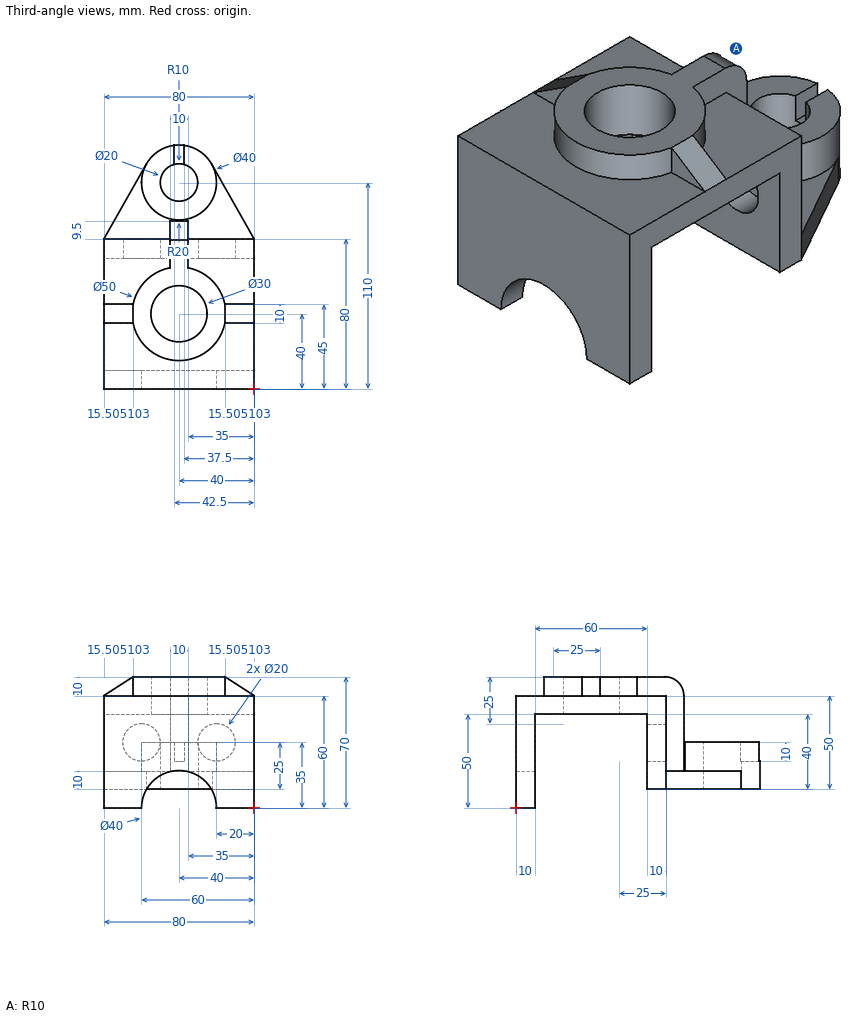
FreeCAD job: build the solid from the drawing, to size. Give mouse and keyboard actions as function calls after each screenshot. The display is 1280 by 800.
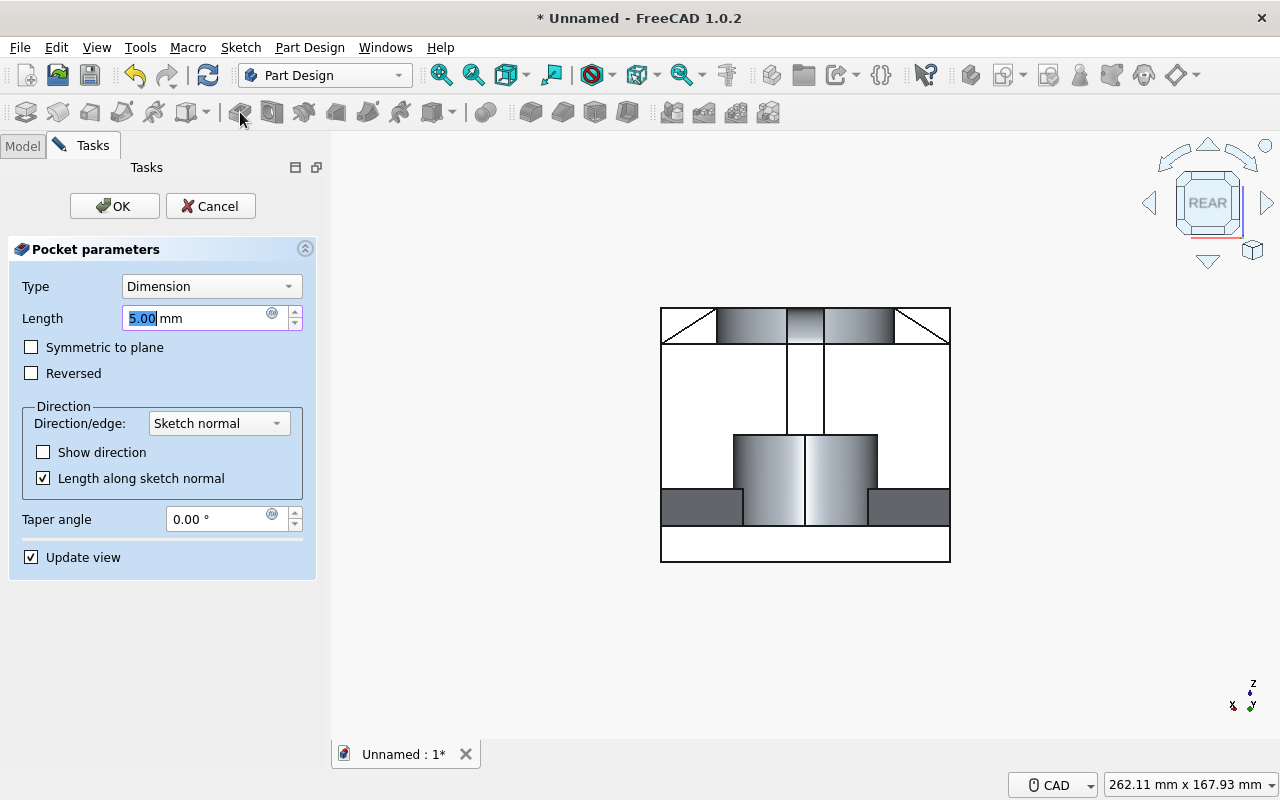
text(25)
key(Tab)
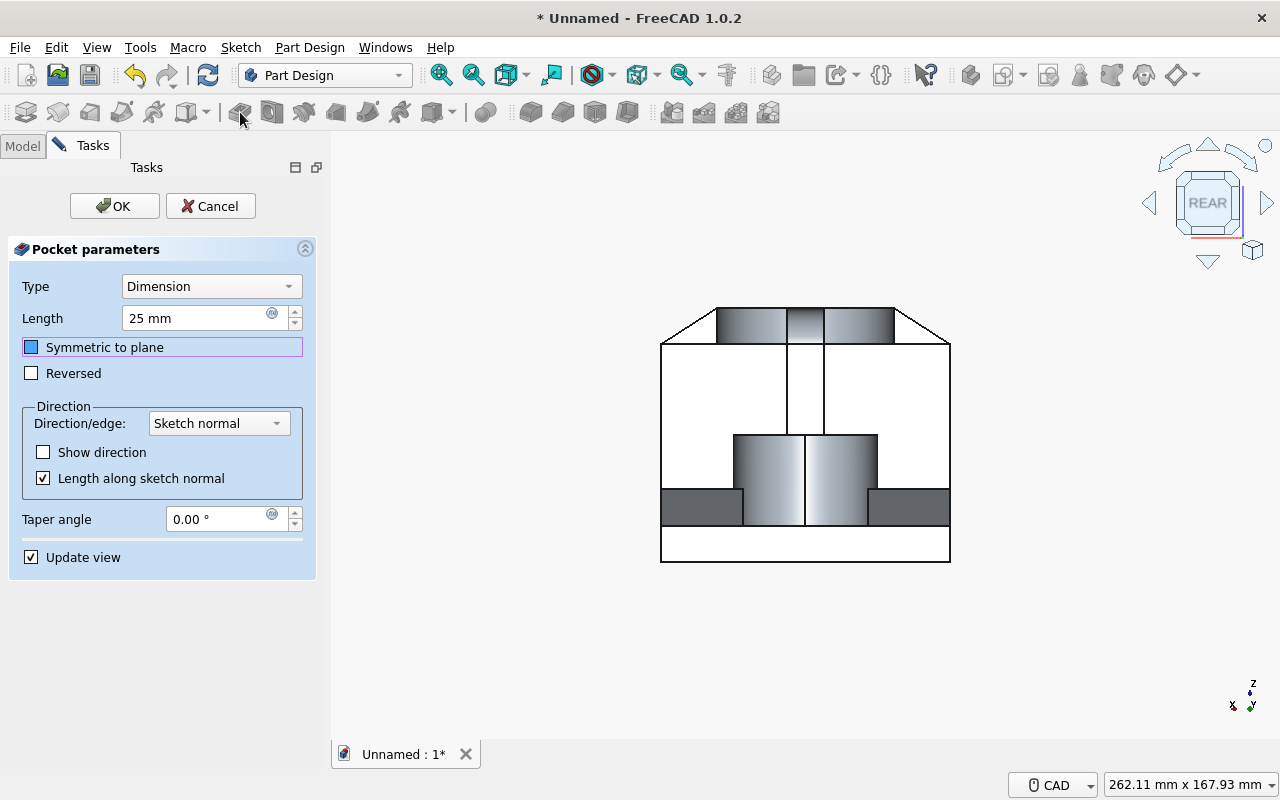
click(115, 206)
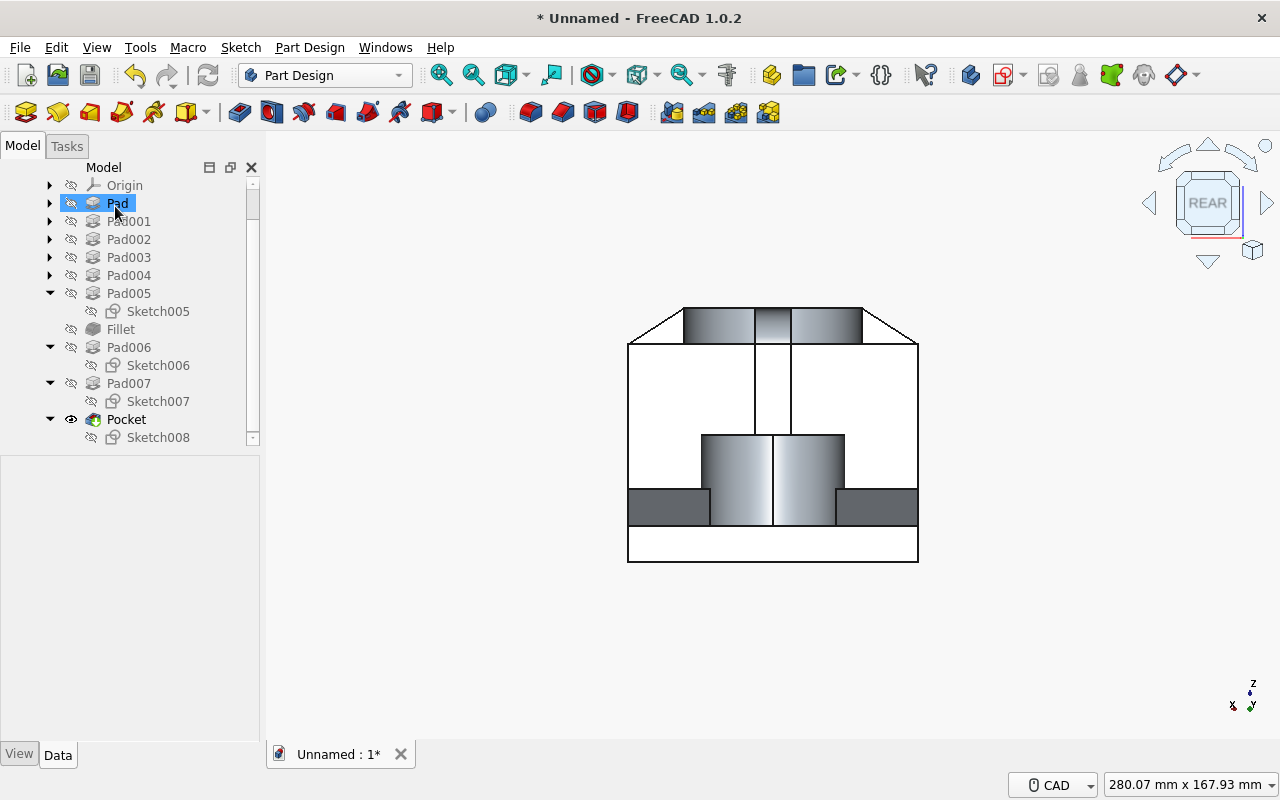
click(442, 76)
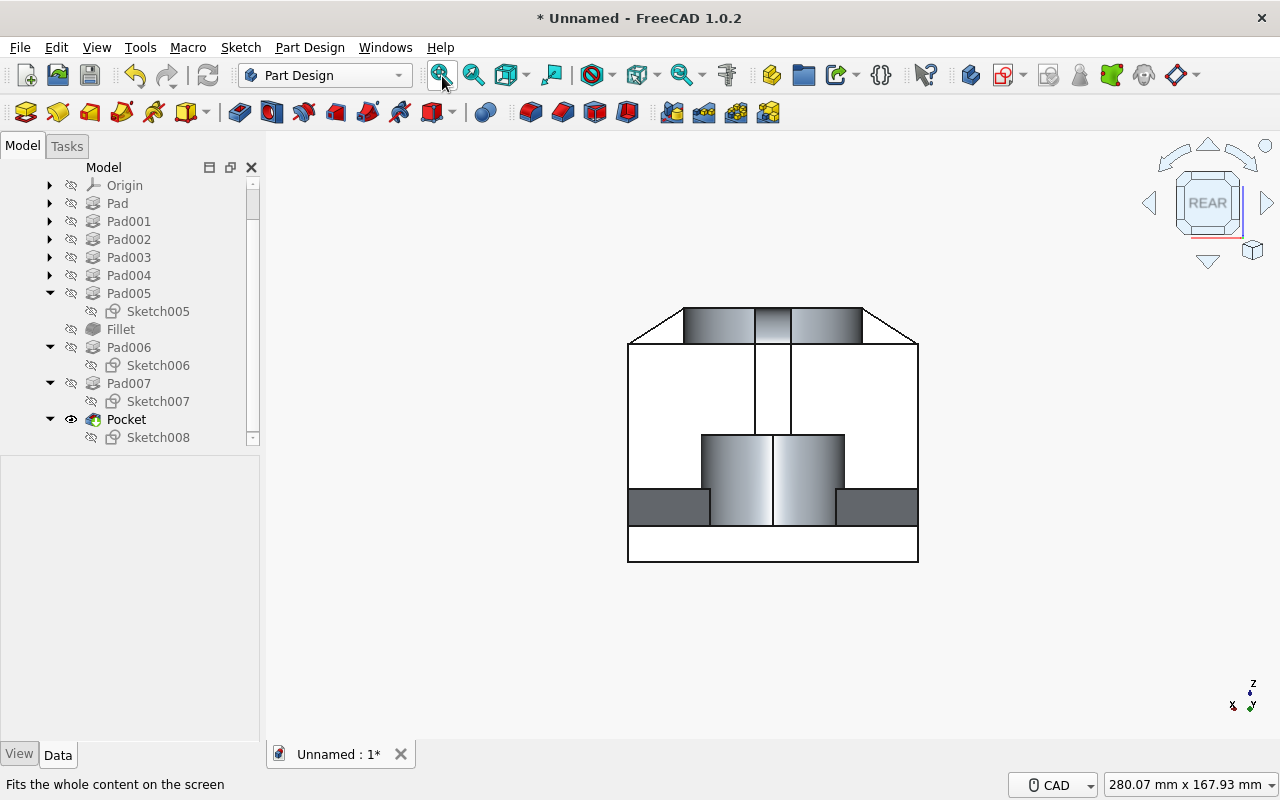
key(0)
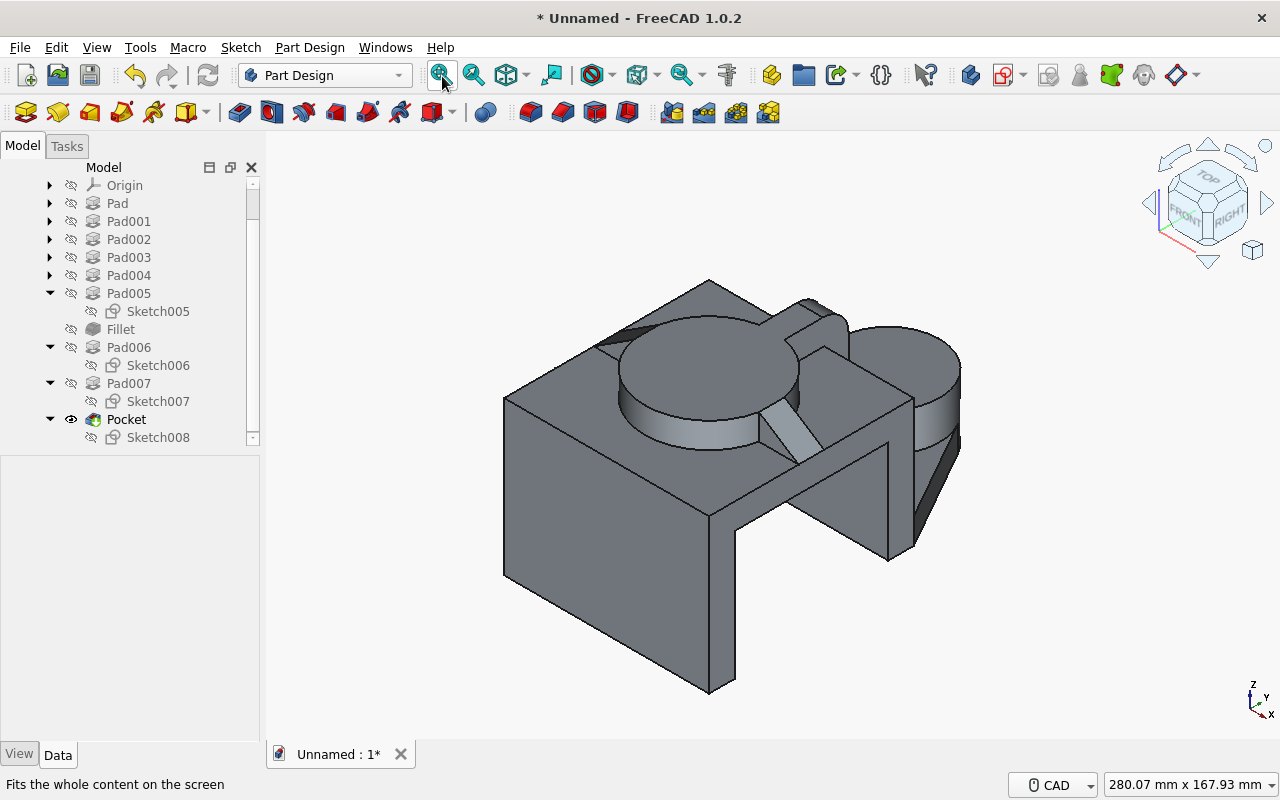
click(704, 370)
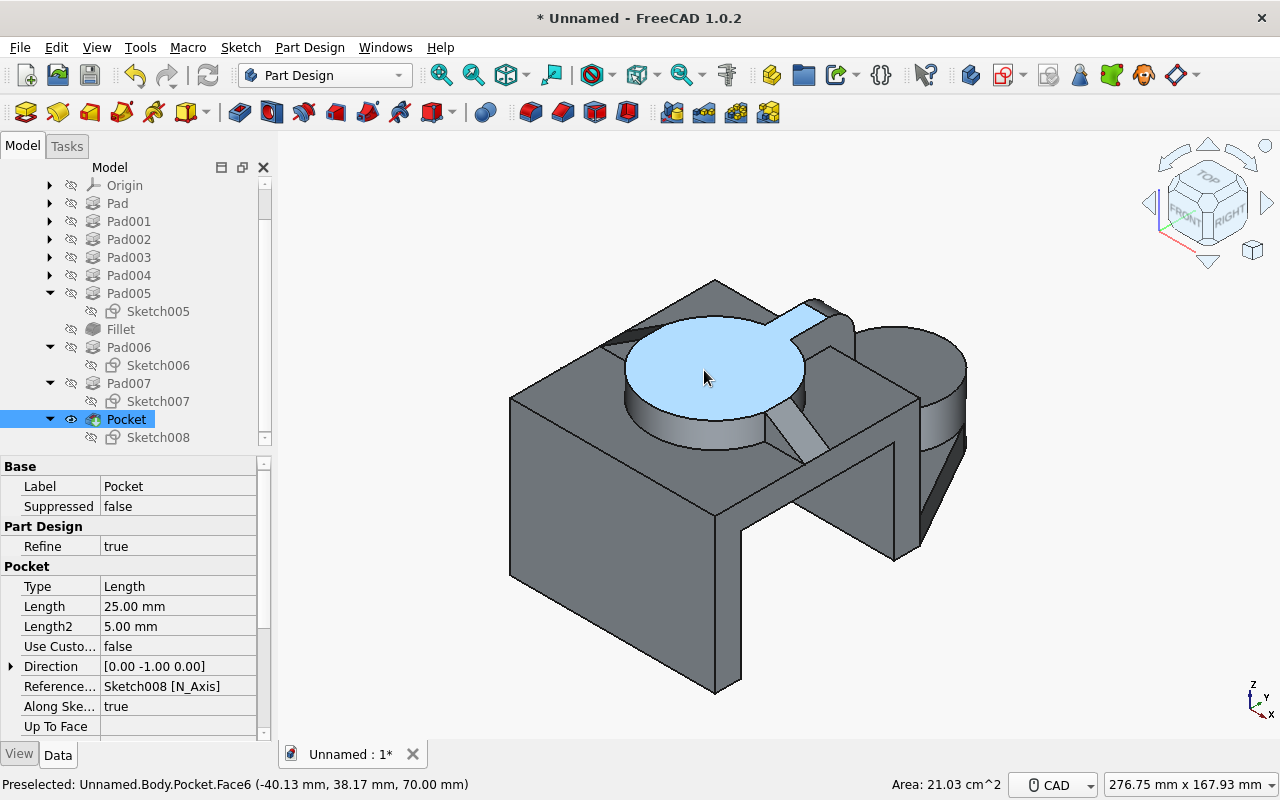
click(1004, 76)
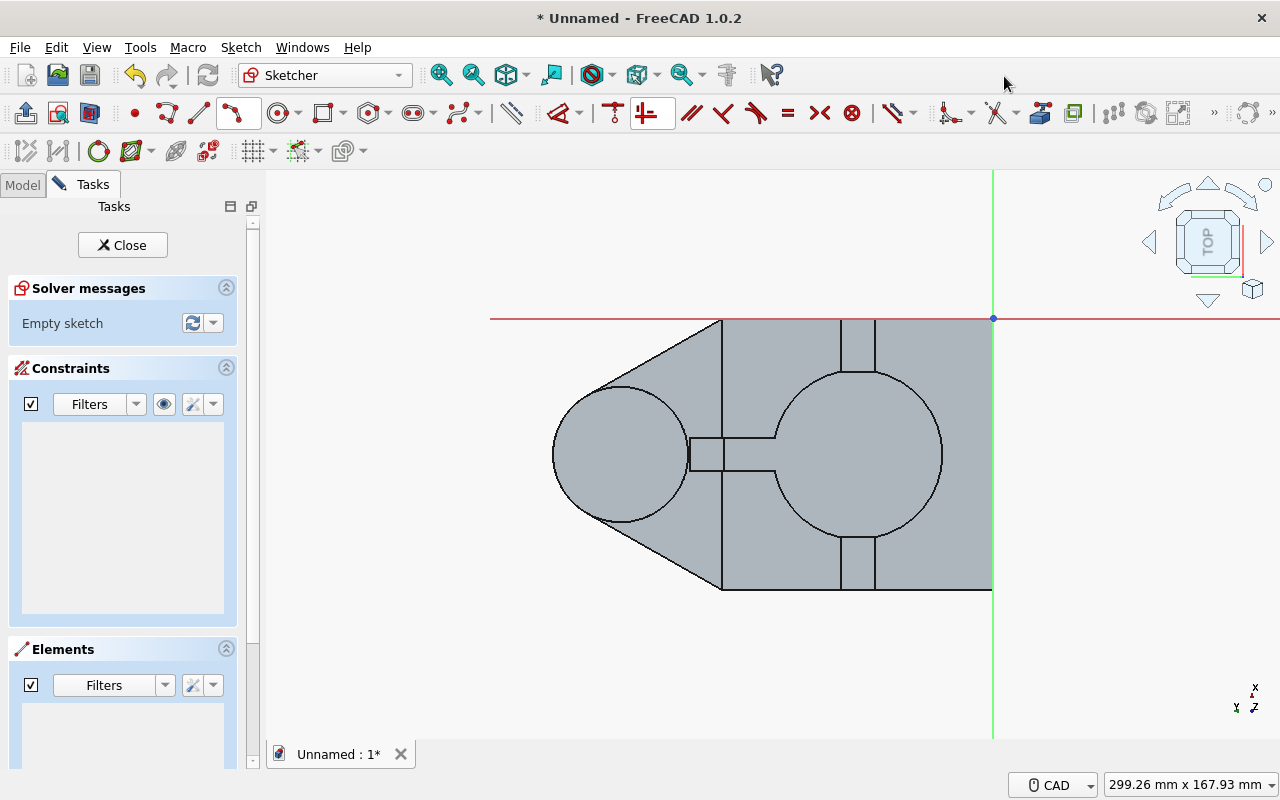
scroll(1115, 361, up, 3)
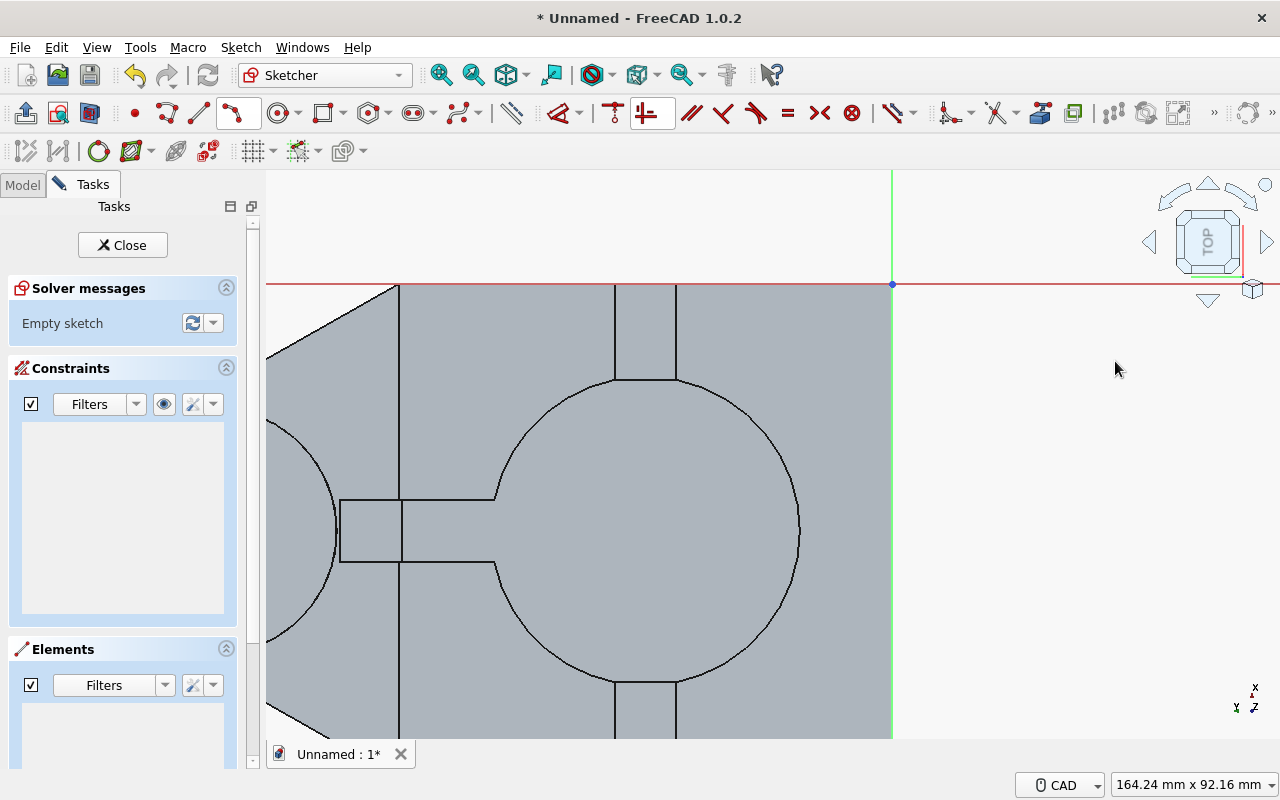
click(278, 114)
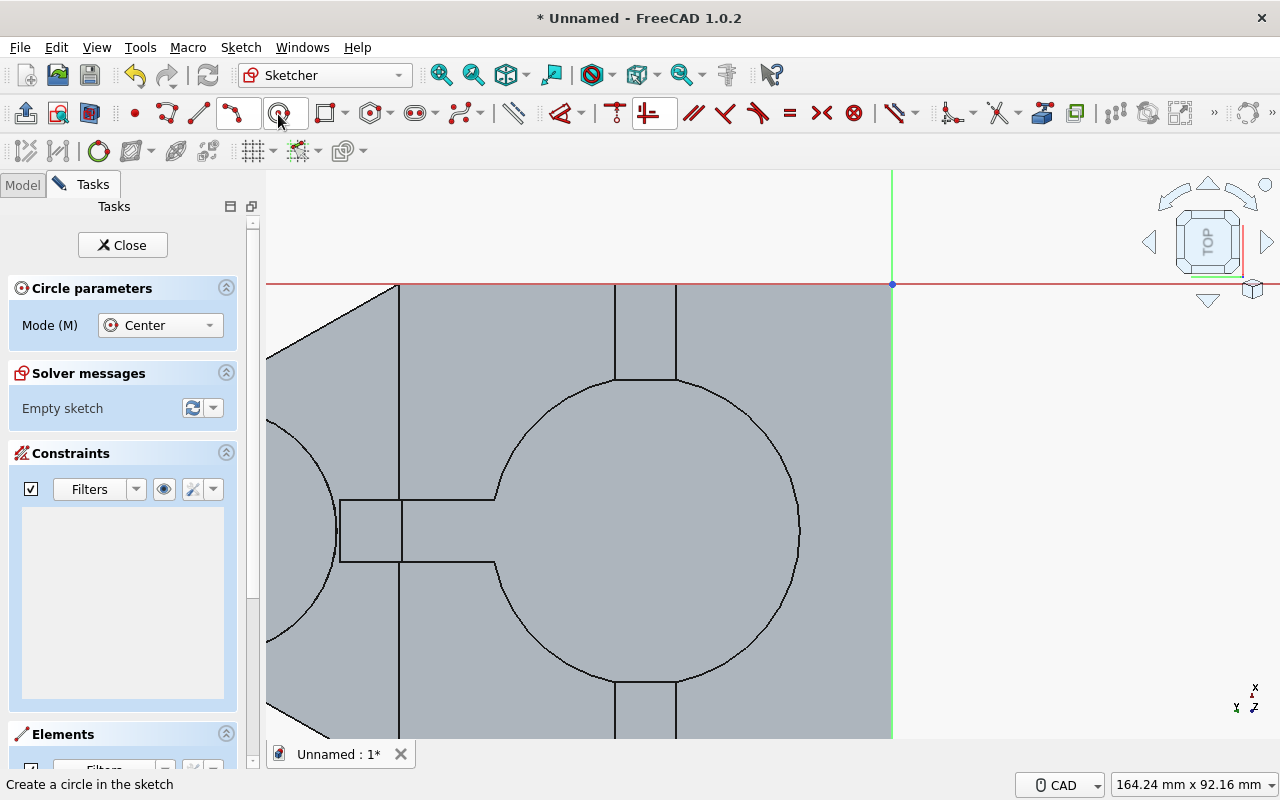
click(645, 531)
move(711, 466)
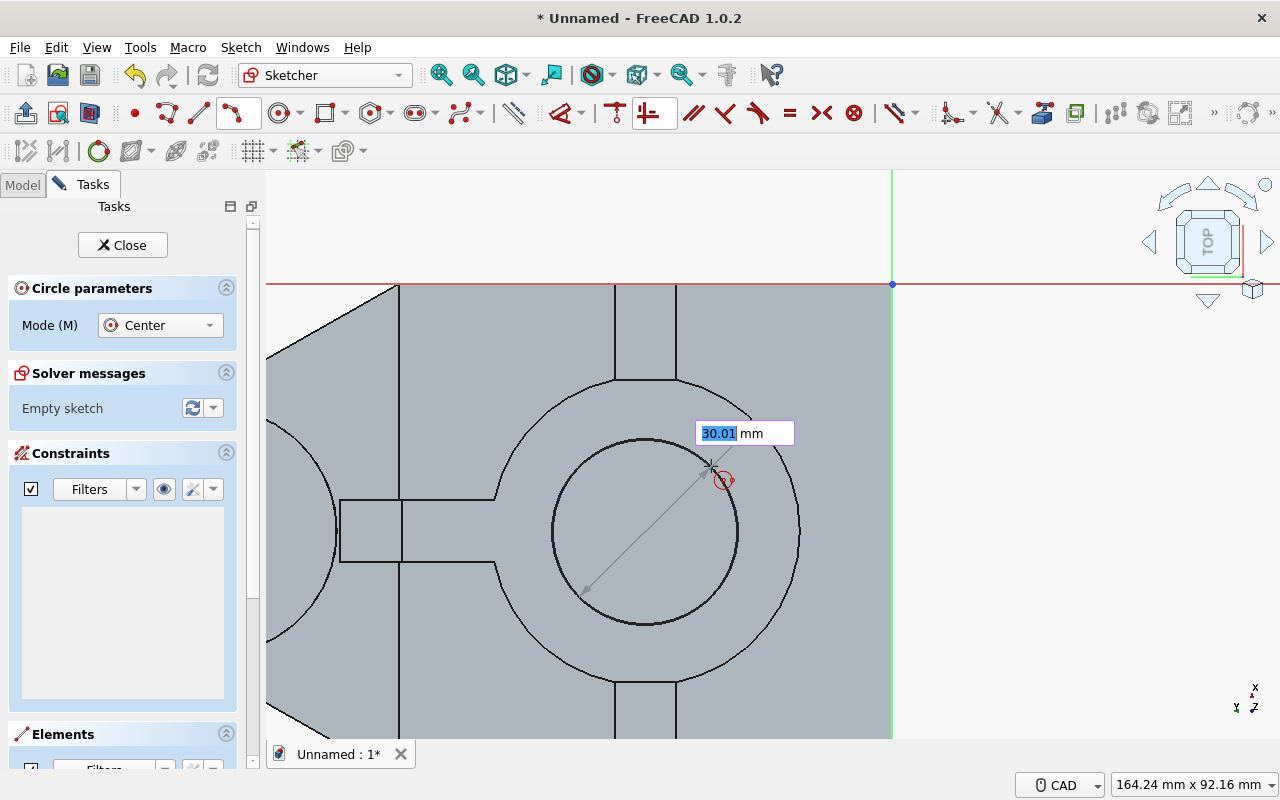
text(30)
key(Return)
key(Escape)